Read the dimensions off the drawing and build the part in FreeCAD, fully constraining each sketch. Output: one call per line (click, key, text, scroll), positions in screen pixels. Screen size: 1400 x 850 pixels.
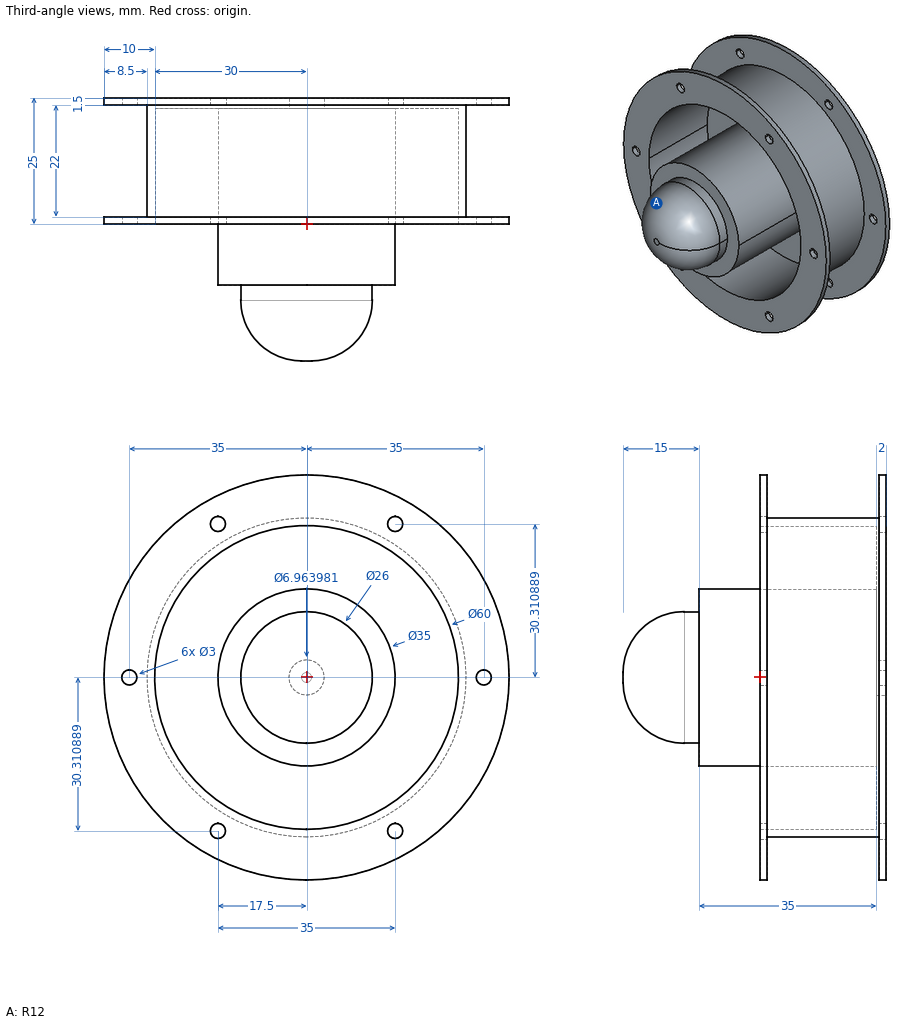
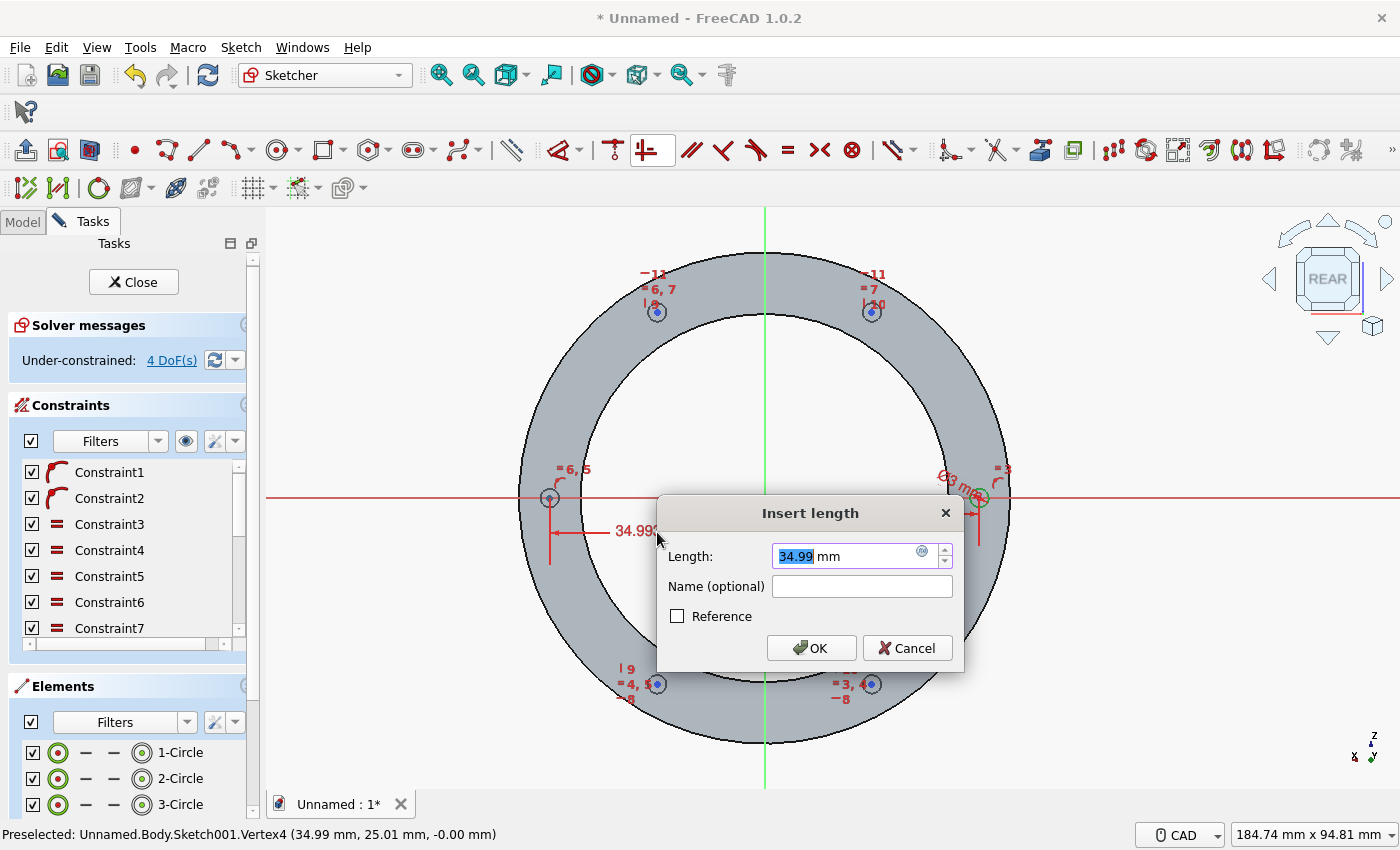
text(35)
key(Return)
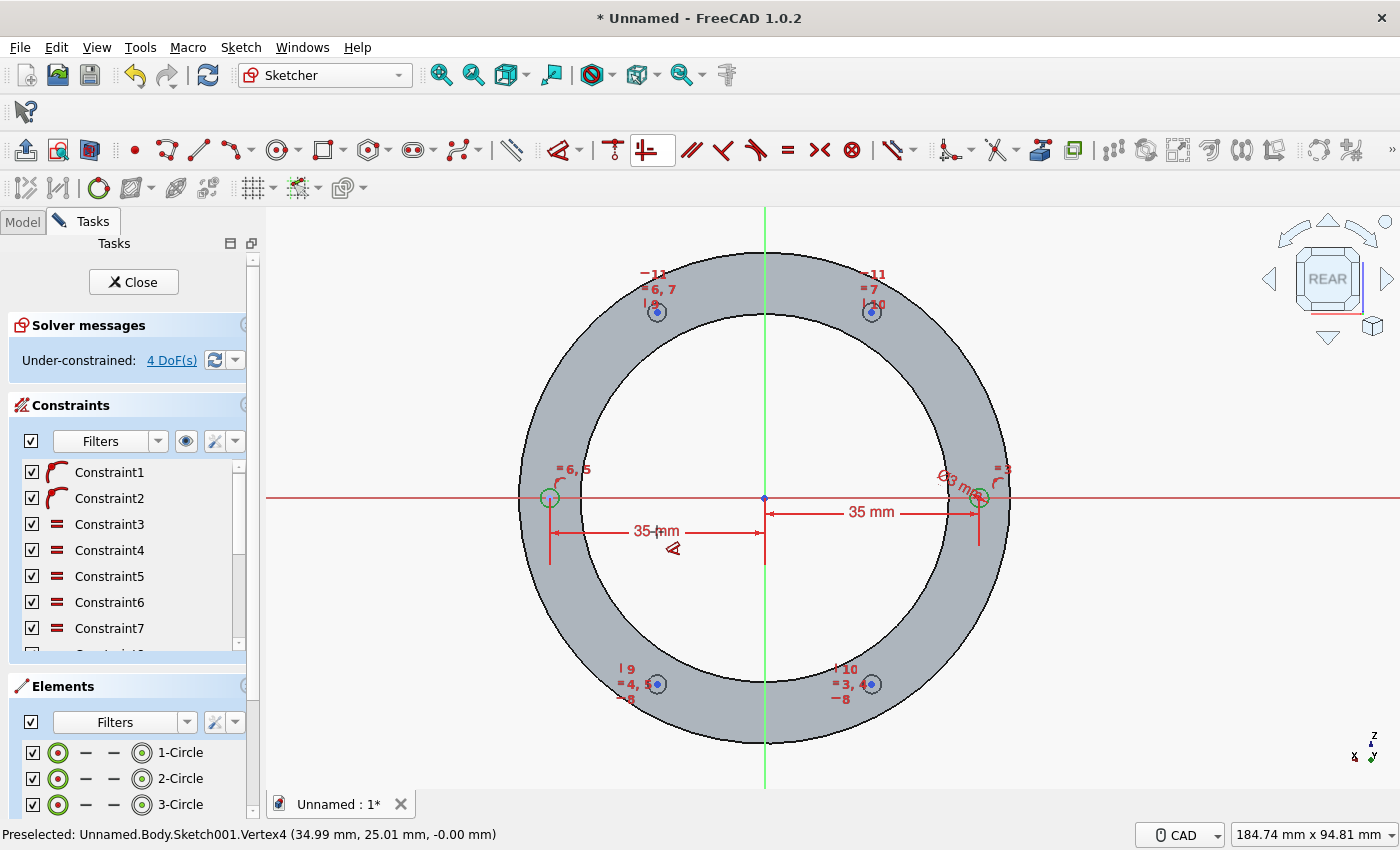
click(872, 684)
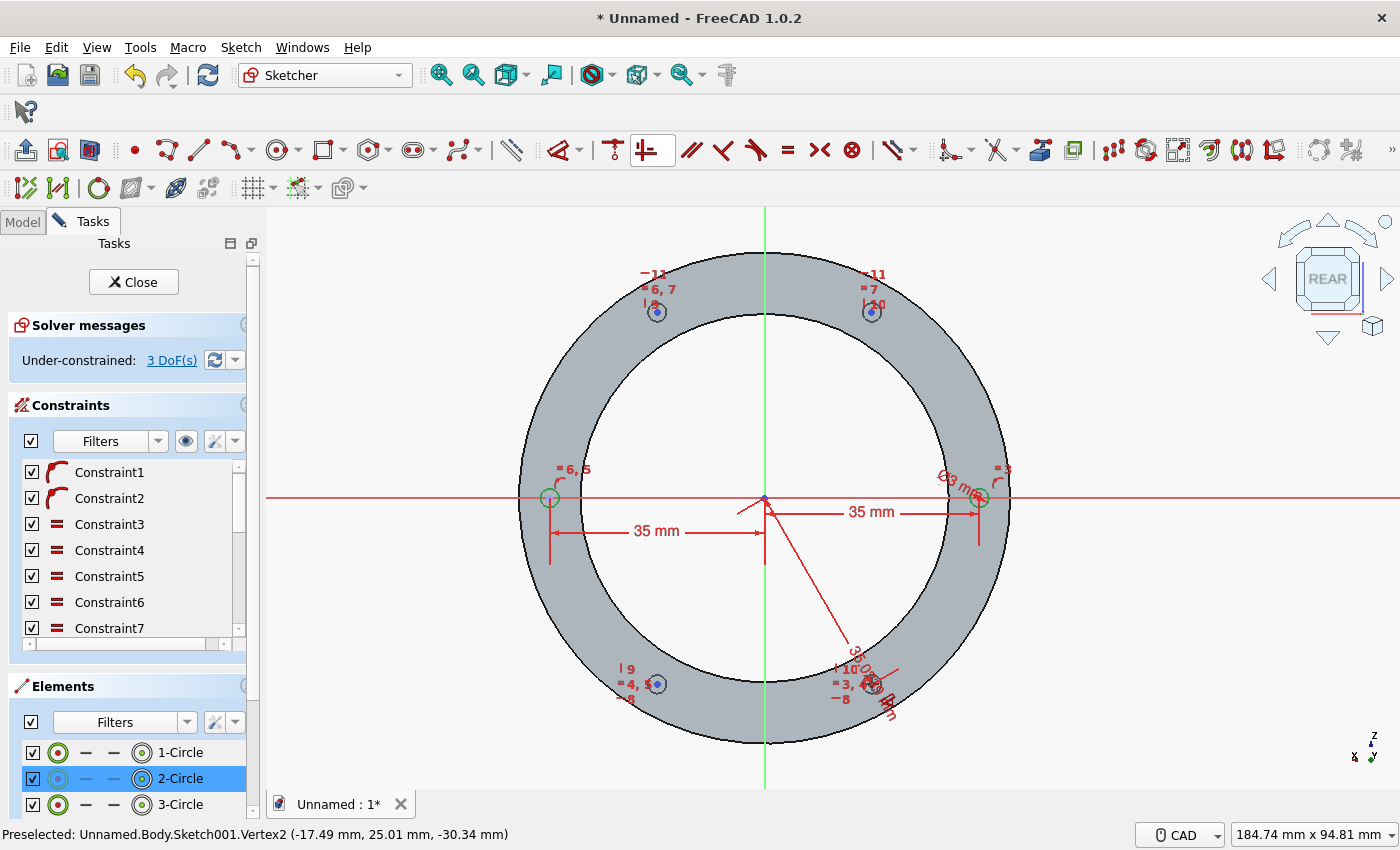
click(657, 684)
click(715, 718)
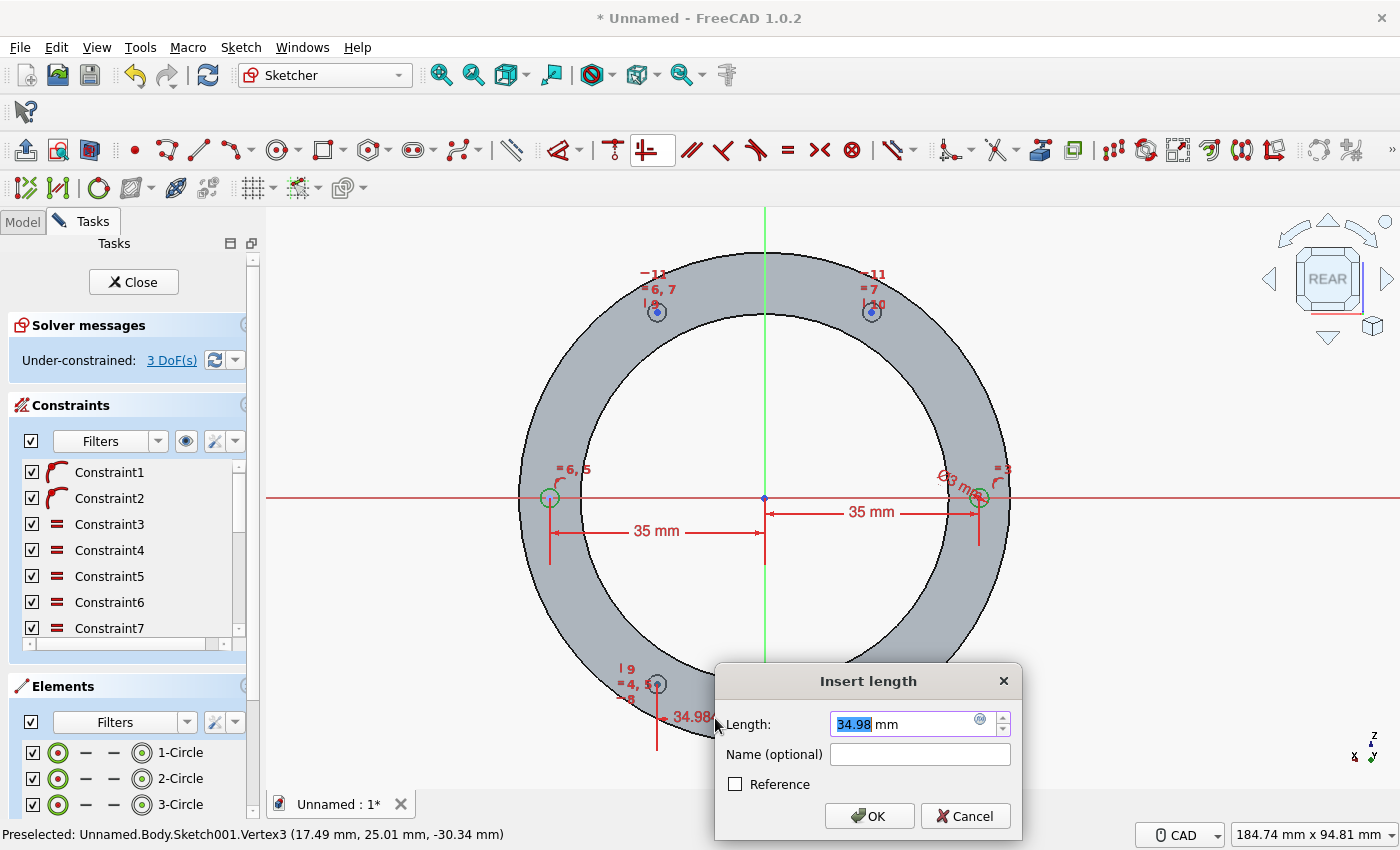
text(35)
key(Return)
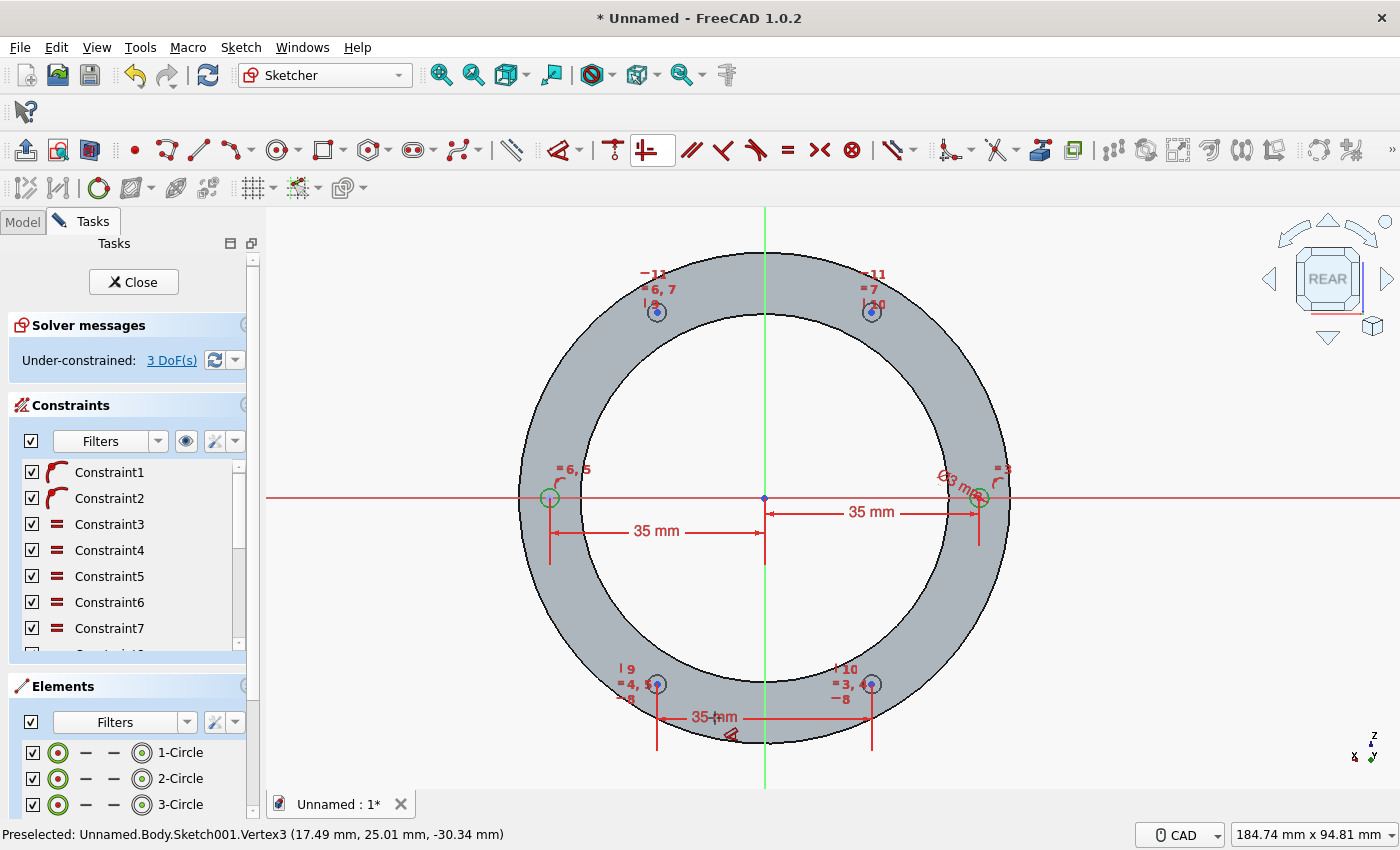
click(872, 684)
click(818, 718)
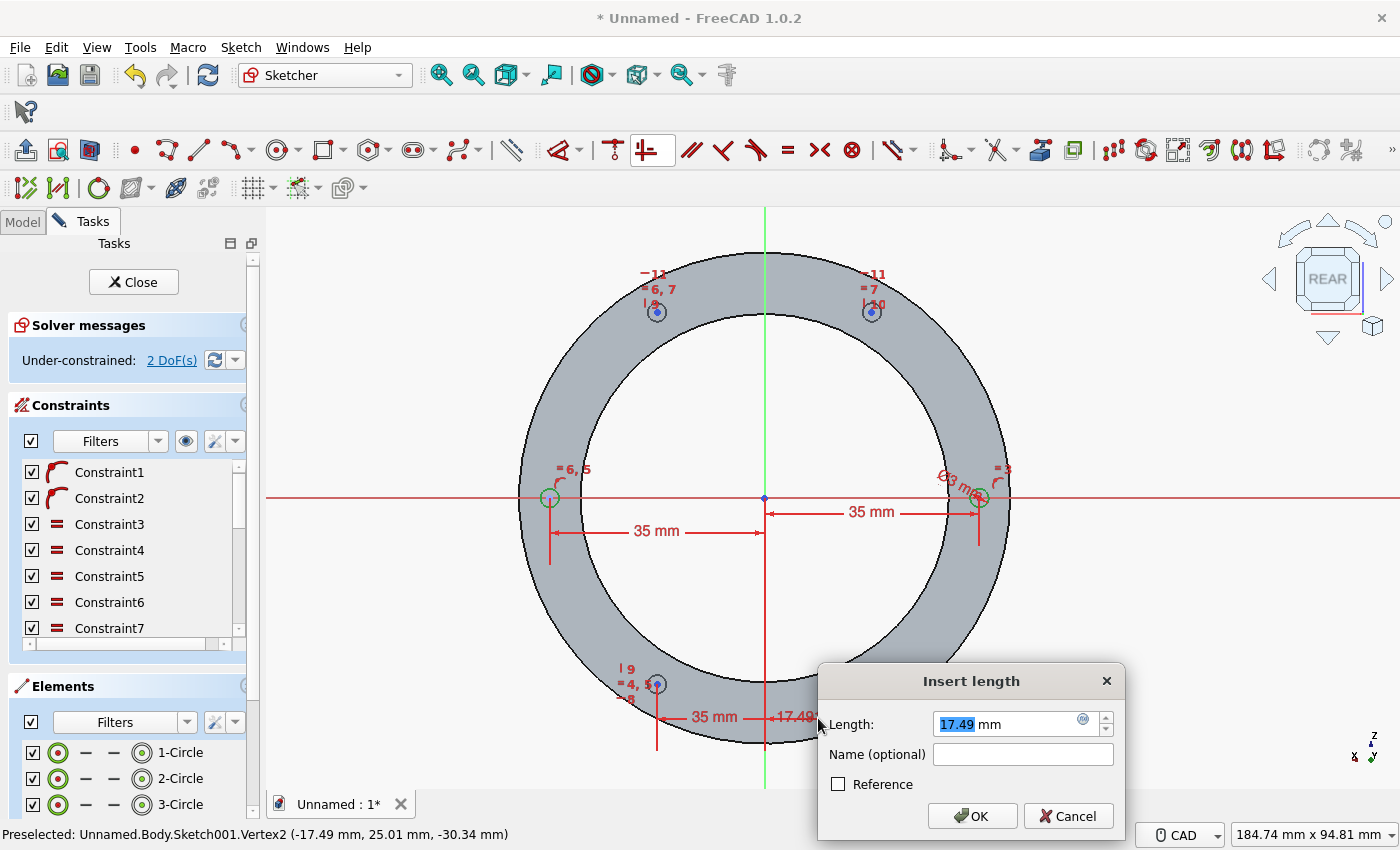
text(17.5)
key(Return)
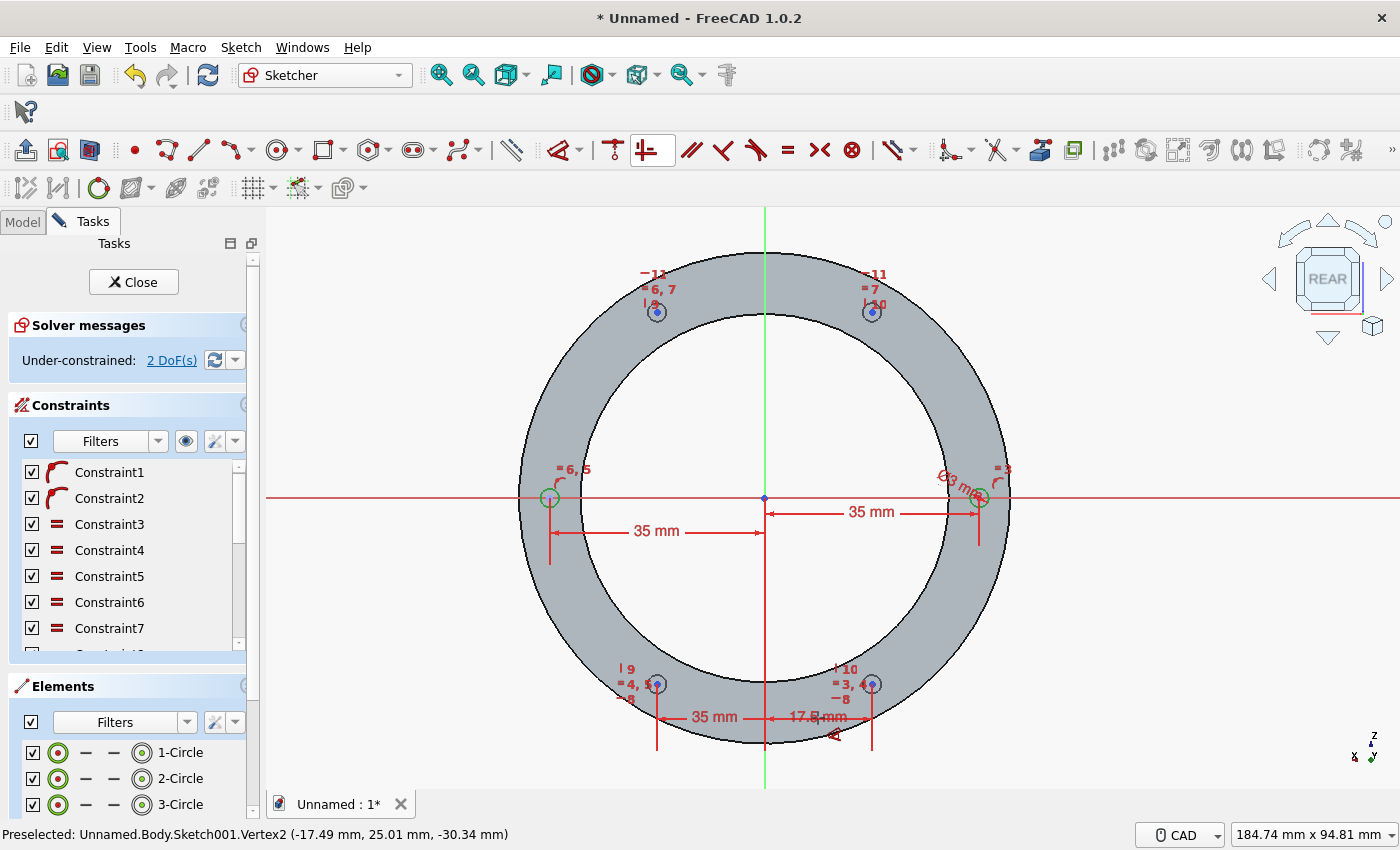
click(872, 684)
click(906, 591)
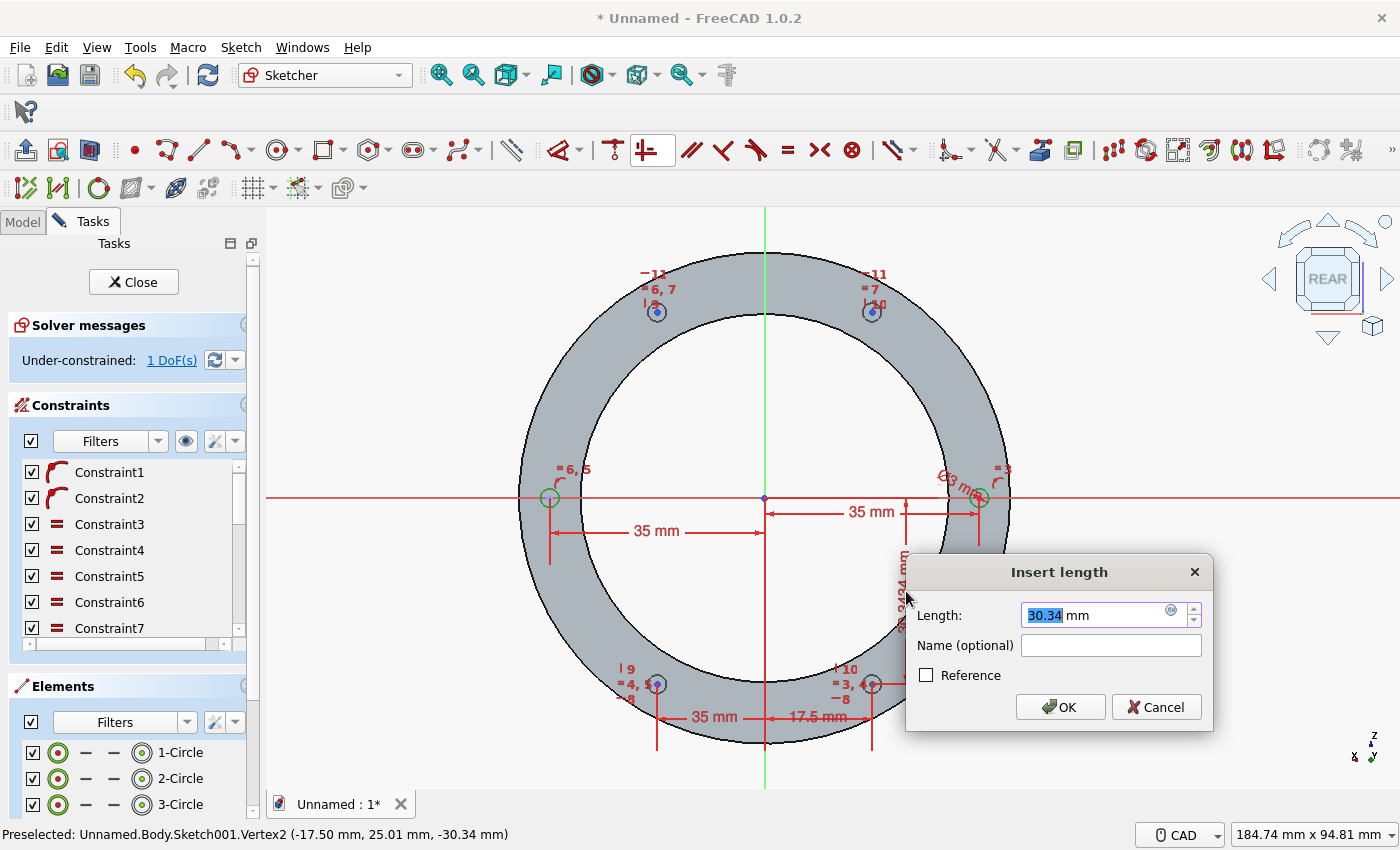
text(30.310889)
key(Return)